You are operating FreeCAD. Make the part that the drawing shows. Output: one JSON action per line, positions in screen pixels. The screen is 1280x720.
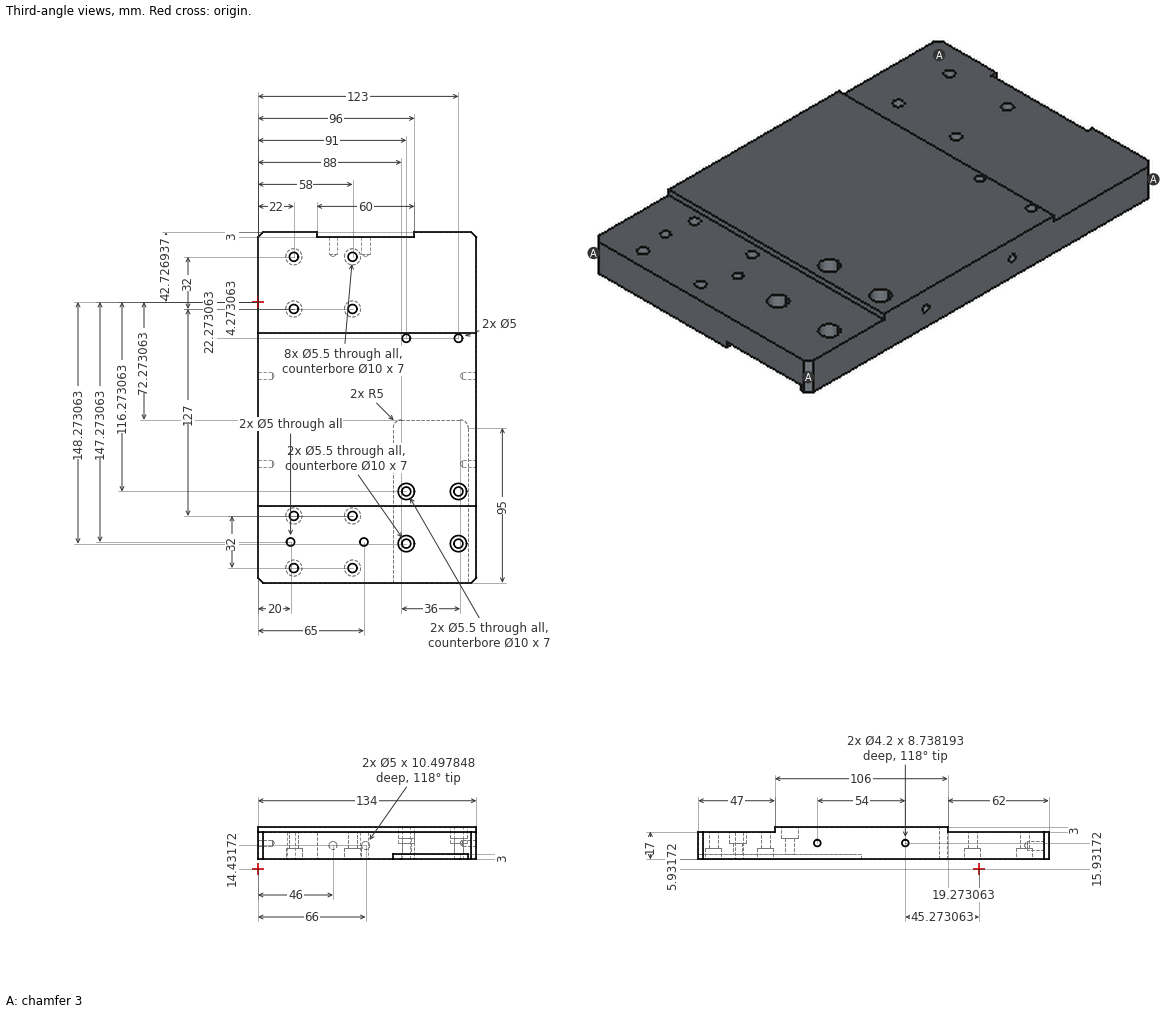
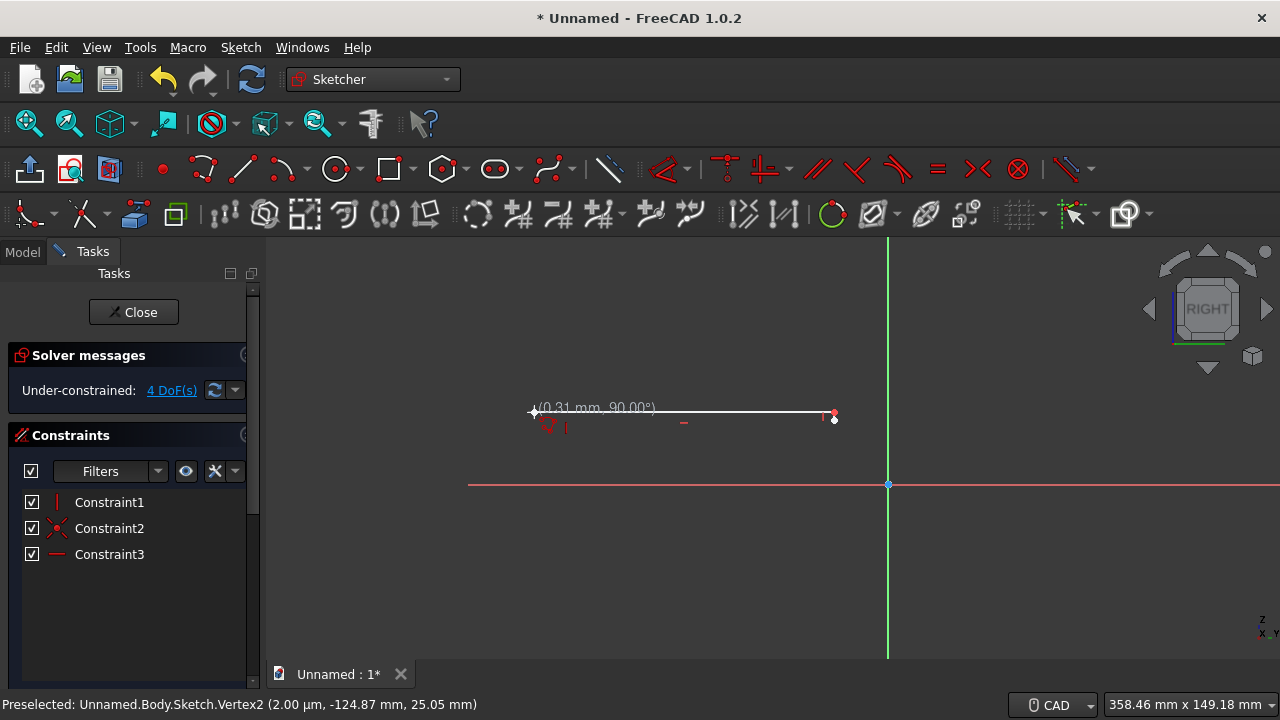
{"action": "scroll", "coordinate": [534, 420], "scroll_direction": "up", "scroll_amount": 4}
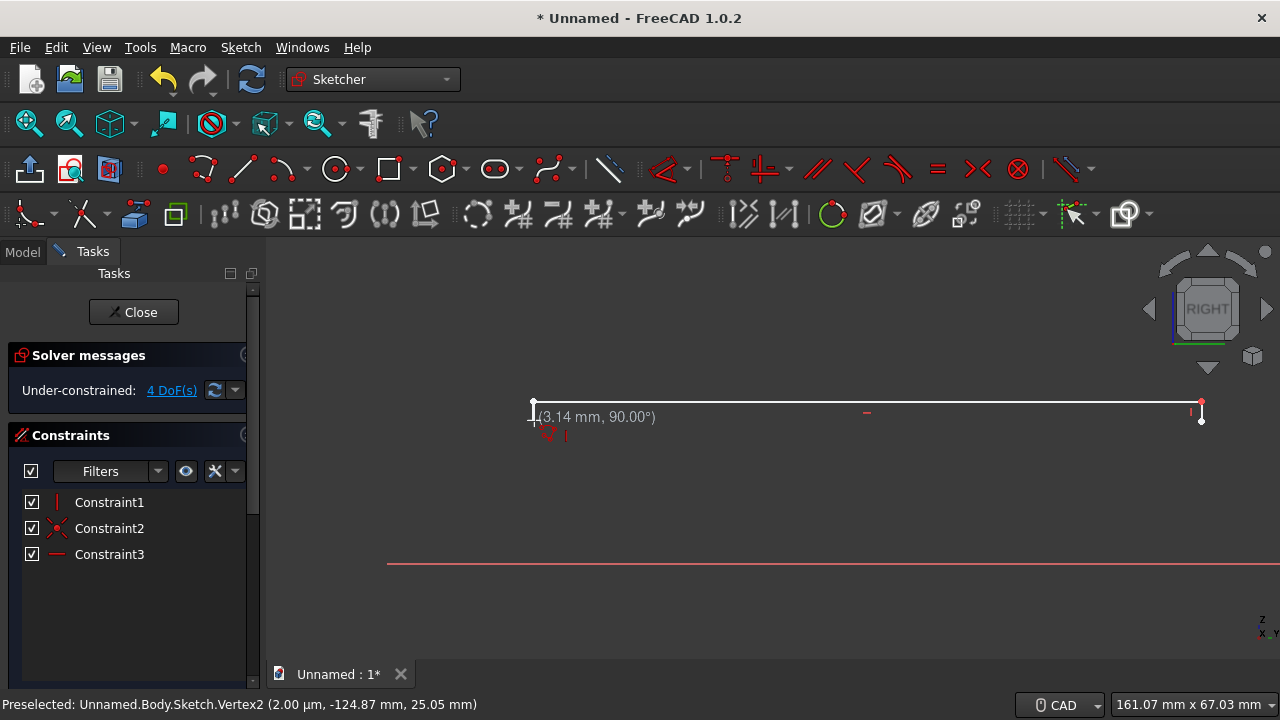
{"action": "left_click", "coordinate": [534, 419]}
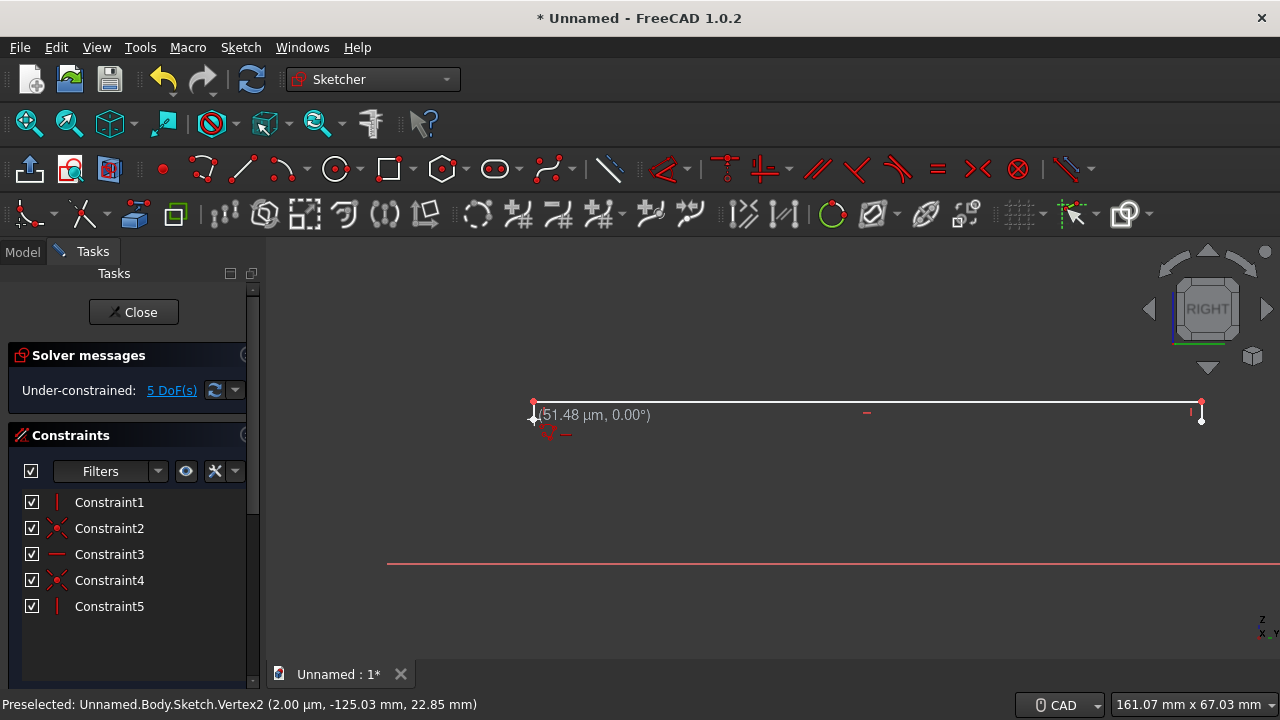
{"action": "scroll", "coordinate": [533, 420], "scroll_direction": "down", "scroll_amount": 4}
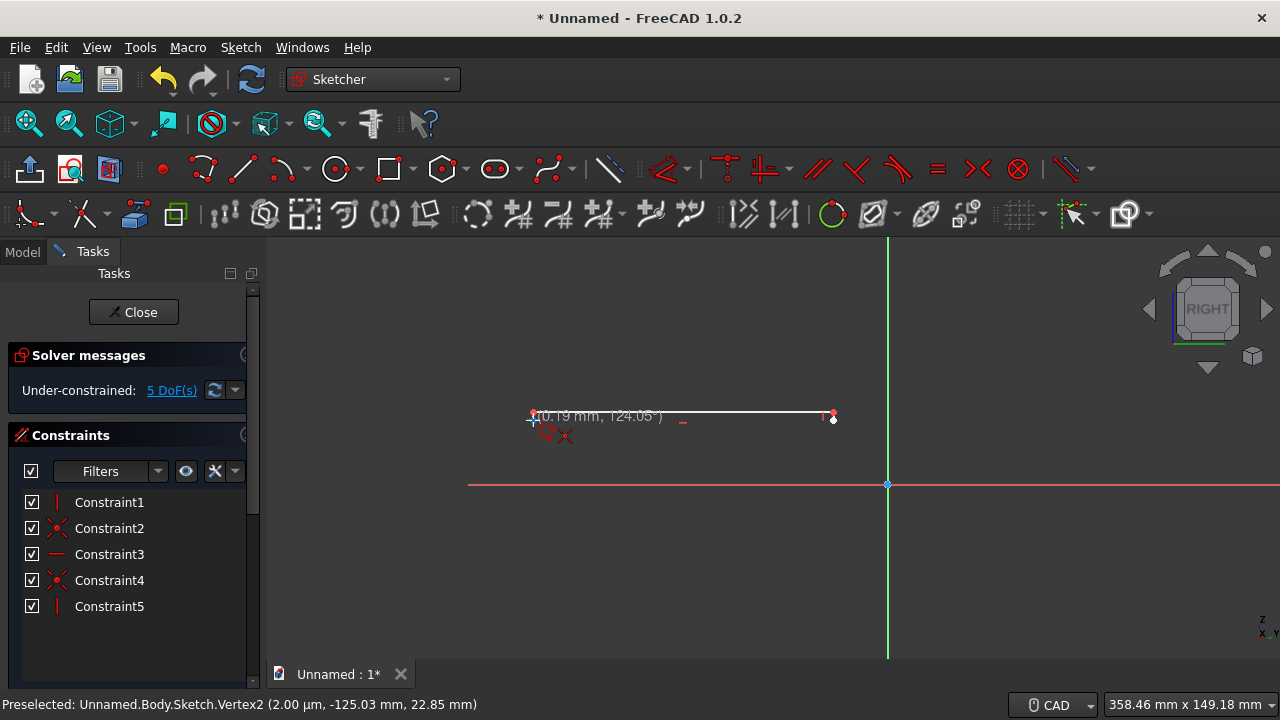
{"action": "left_click", "coordinate": [400, 420]}
{"action": "left_click", "coordinate": [400, 468]}
{"action": "left_click", "coordinate": [1009, 468]}
{"action": "left_click", "coordinate": [1009, 420]}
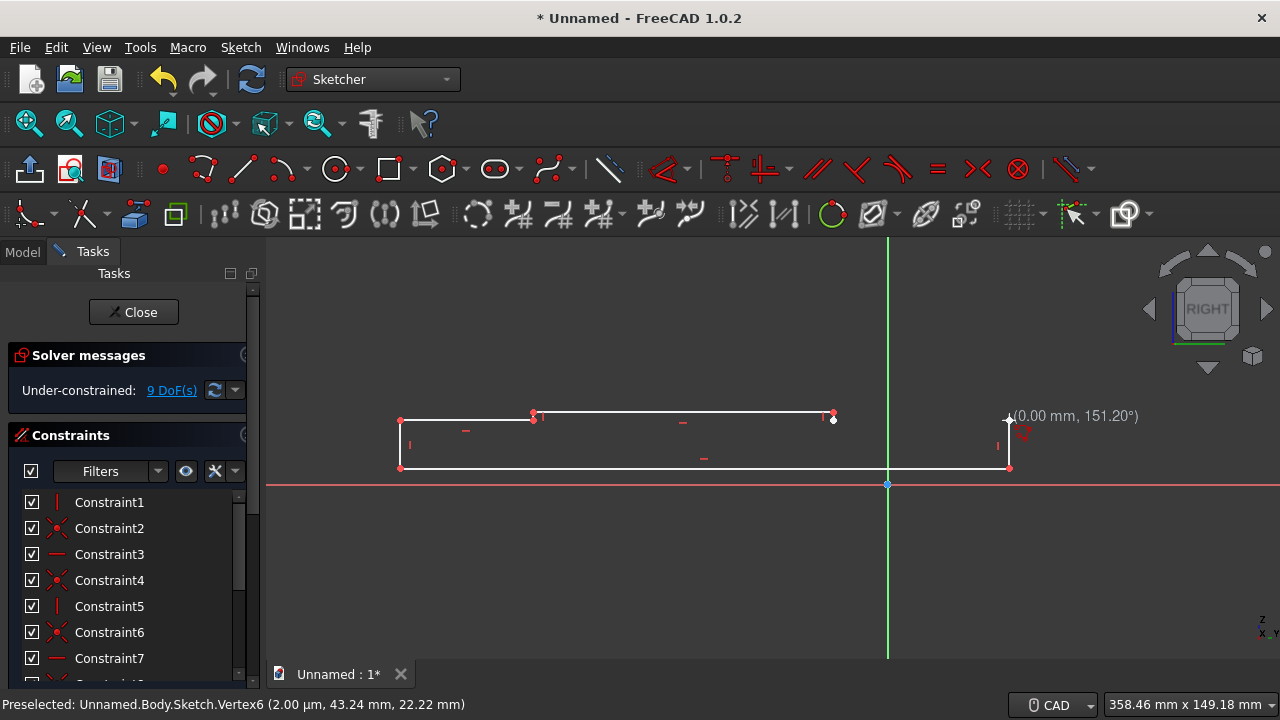
{"action": "scroll", "coordinate": [833, 420], "scroll_direction": "up", "scroll_amount": 7}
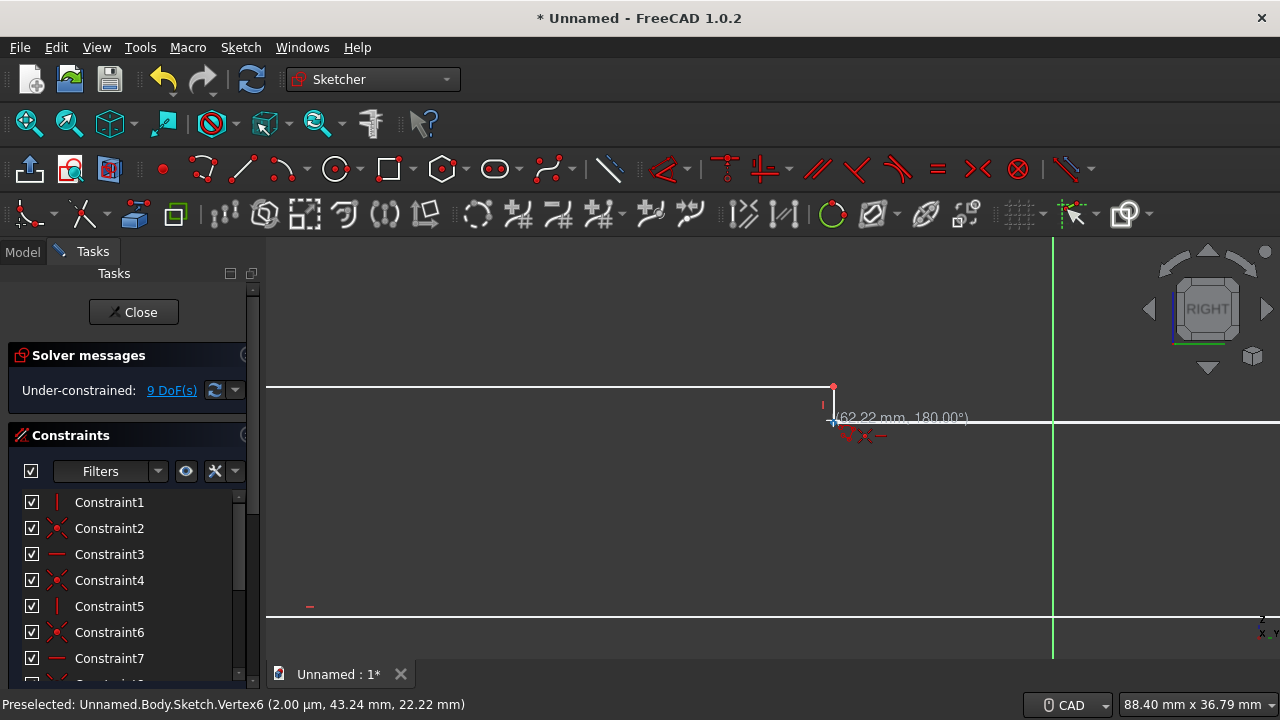
{"action": "left_click", "coordinate": [834, 423]}
{"action": "key", "text": "Escape"}
{"action": "key", "text": "Escape"}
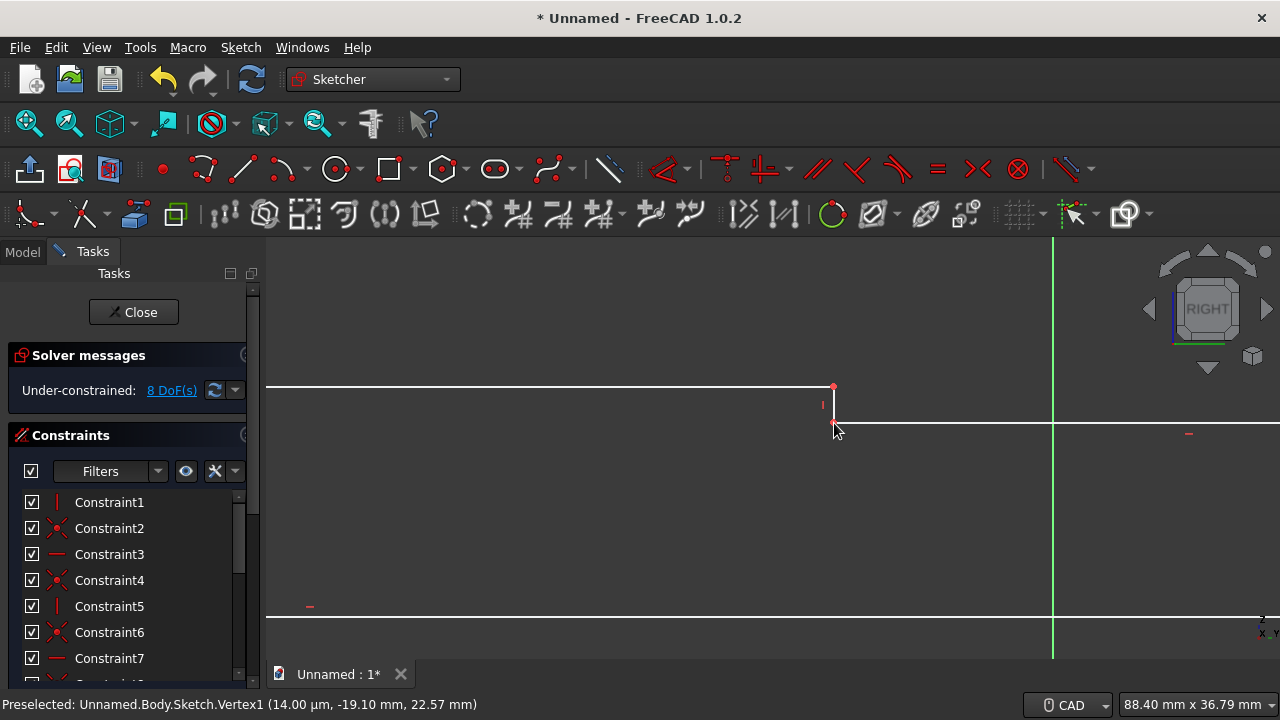
{"action": "left_click", "coordinate": [664, 170]}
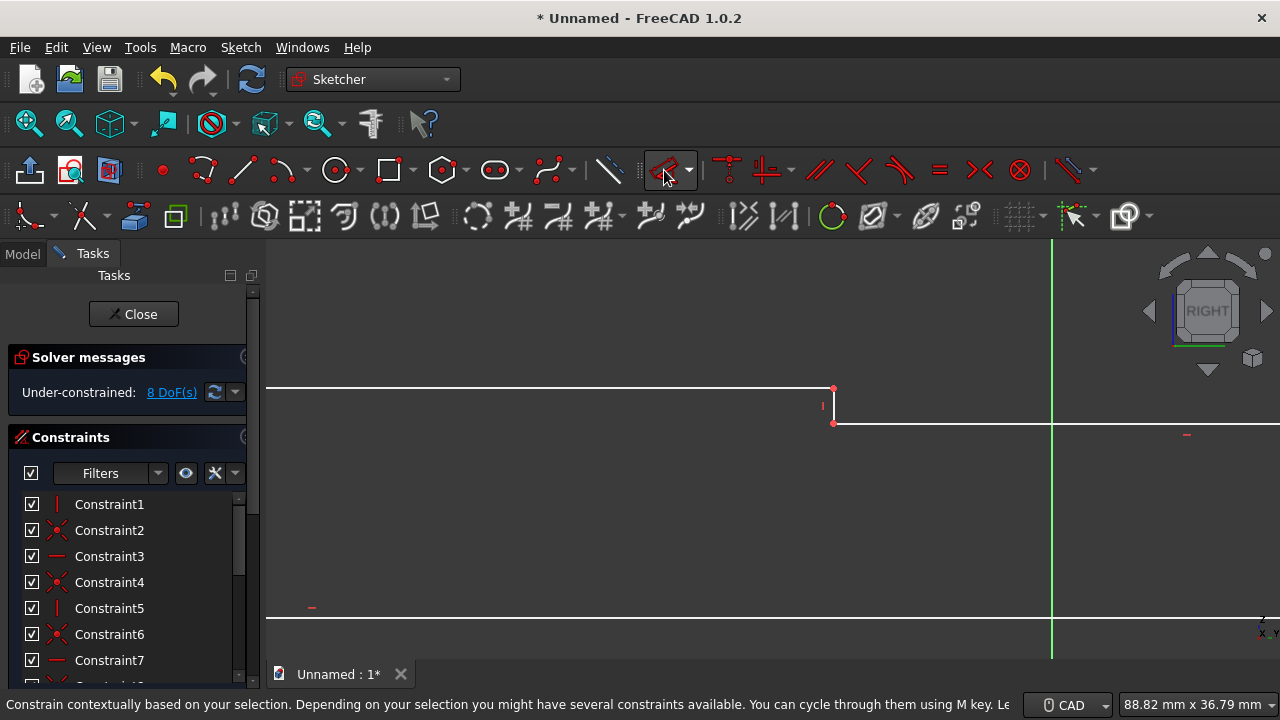
{"action": "scroll", "coordinate": [834, 413], "scroll_direction": "up", "scroll_amount": 2}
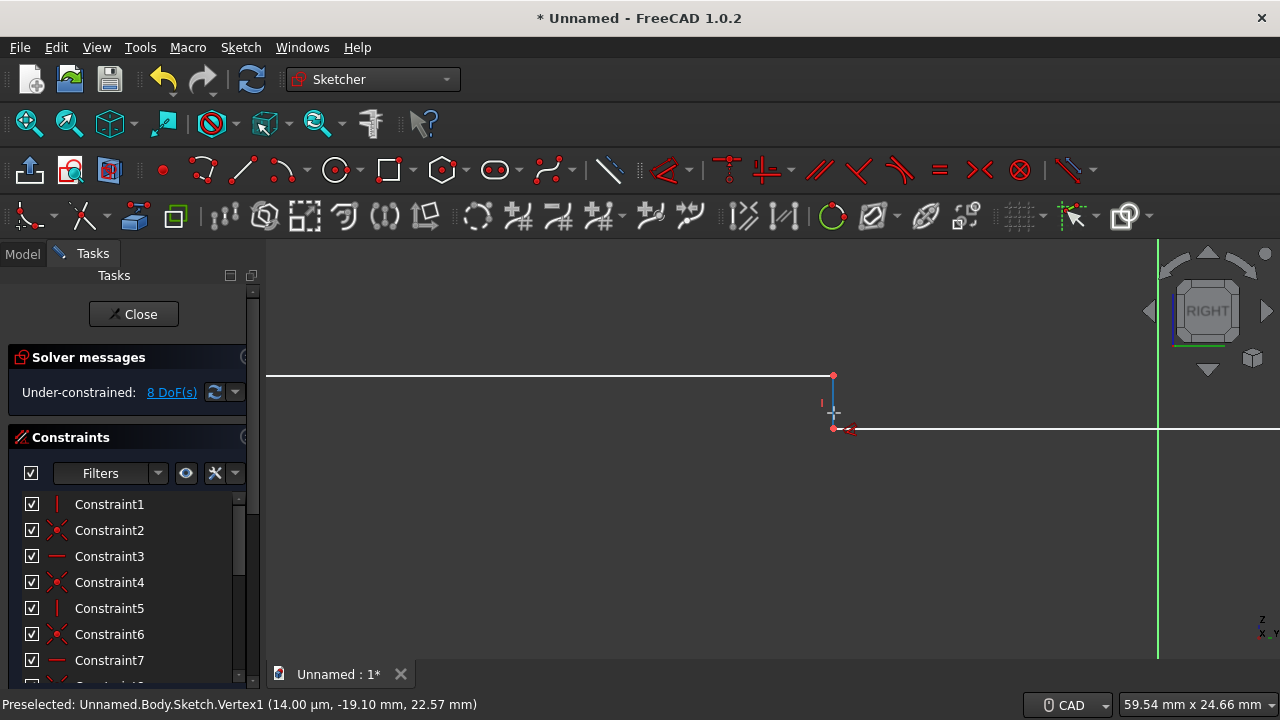
{"action": "left_click", "coordinate": [833, 413]}
{"action": "left_click", "coordinate": [867, 402]}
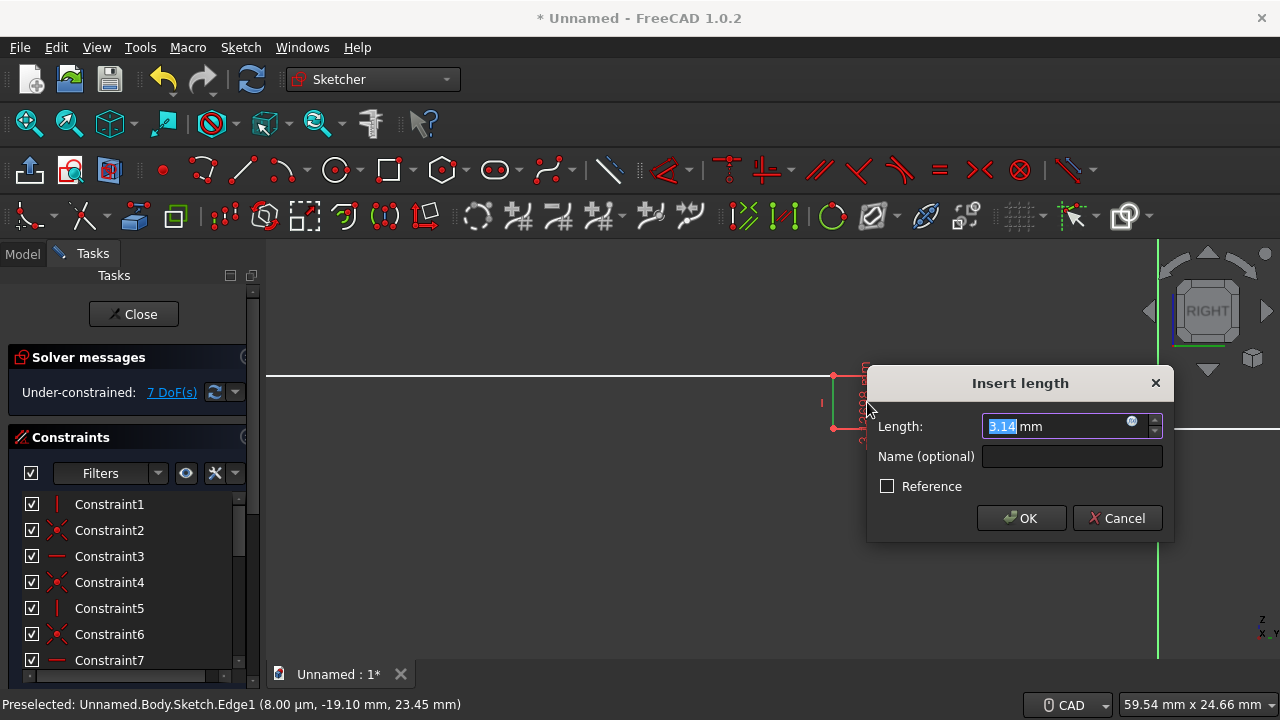
{"action": "type", "text": "3"}
{"action": "key", "text": "Return"}